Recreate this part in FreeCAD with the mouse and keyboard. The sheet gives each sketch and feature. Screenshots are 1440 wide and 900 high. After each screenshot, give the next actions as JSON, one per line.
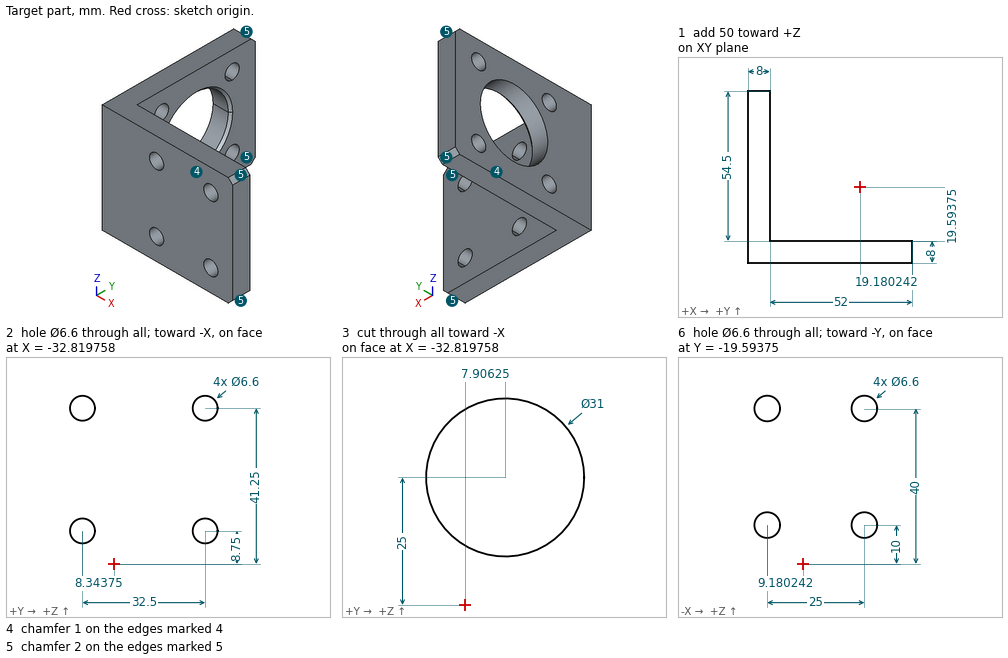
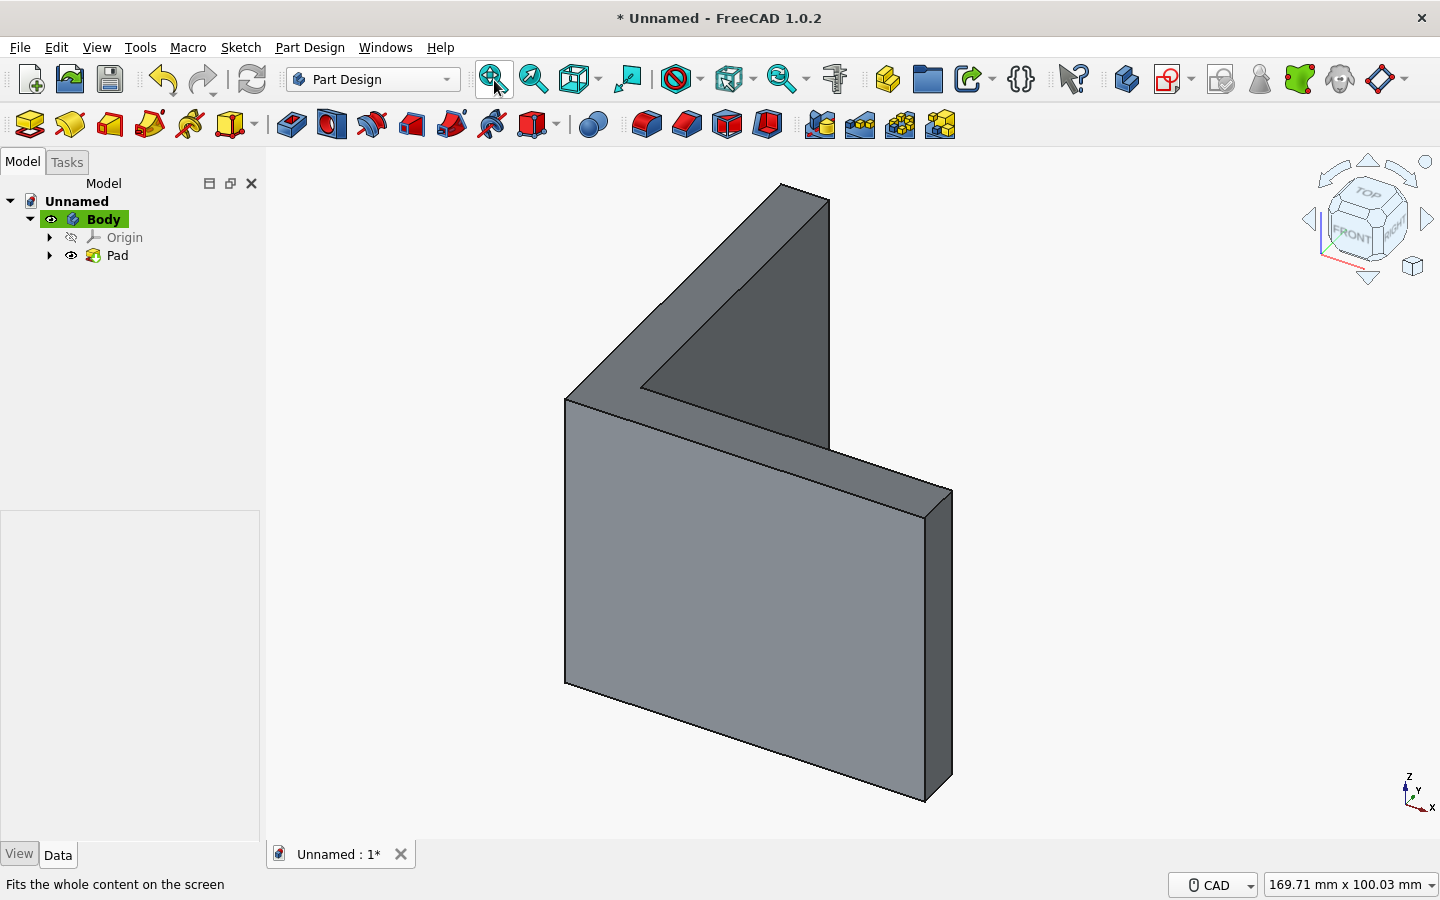
{"action": "left_click", "coordinate": [762, 408]}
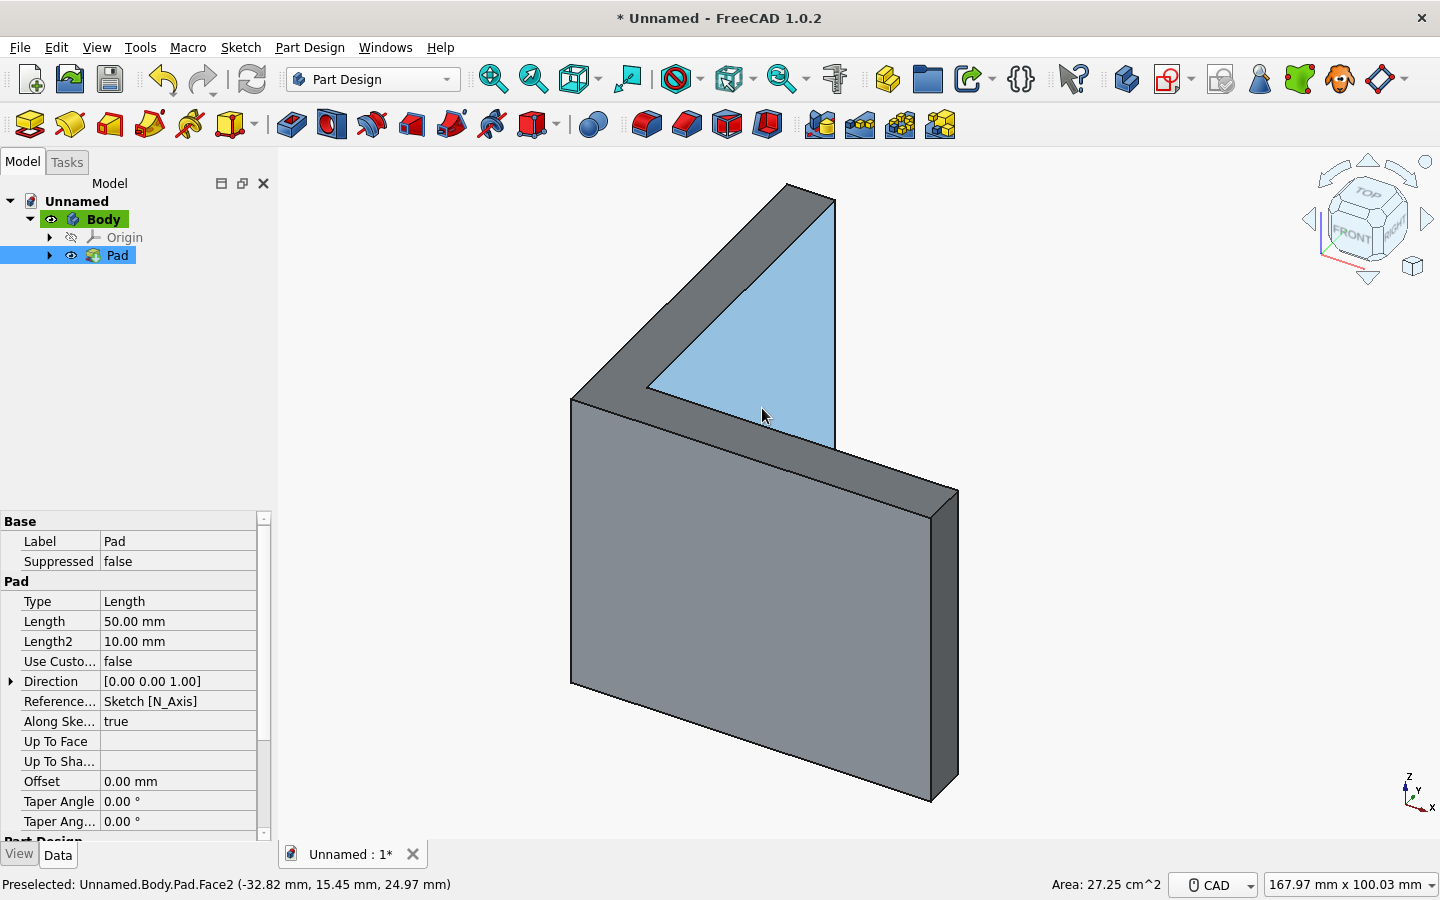
{"action": "left_click", "coordinate": [1168, 80]}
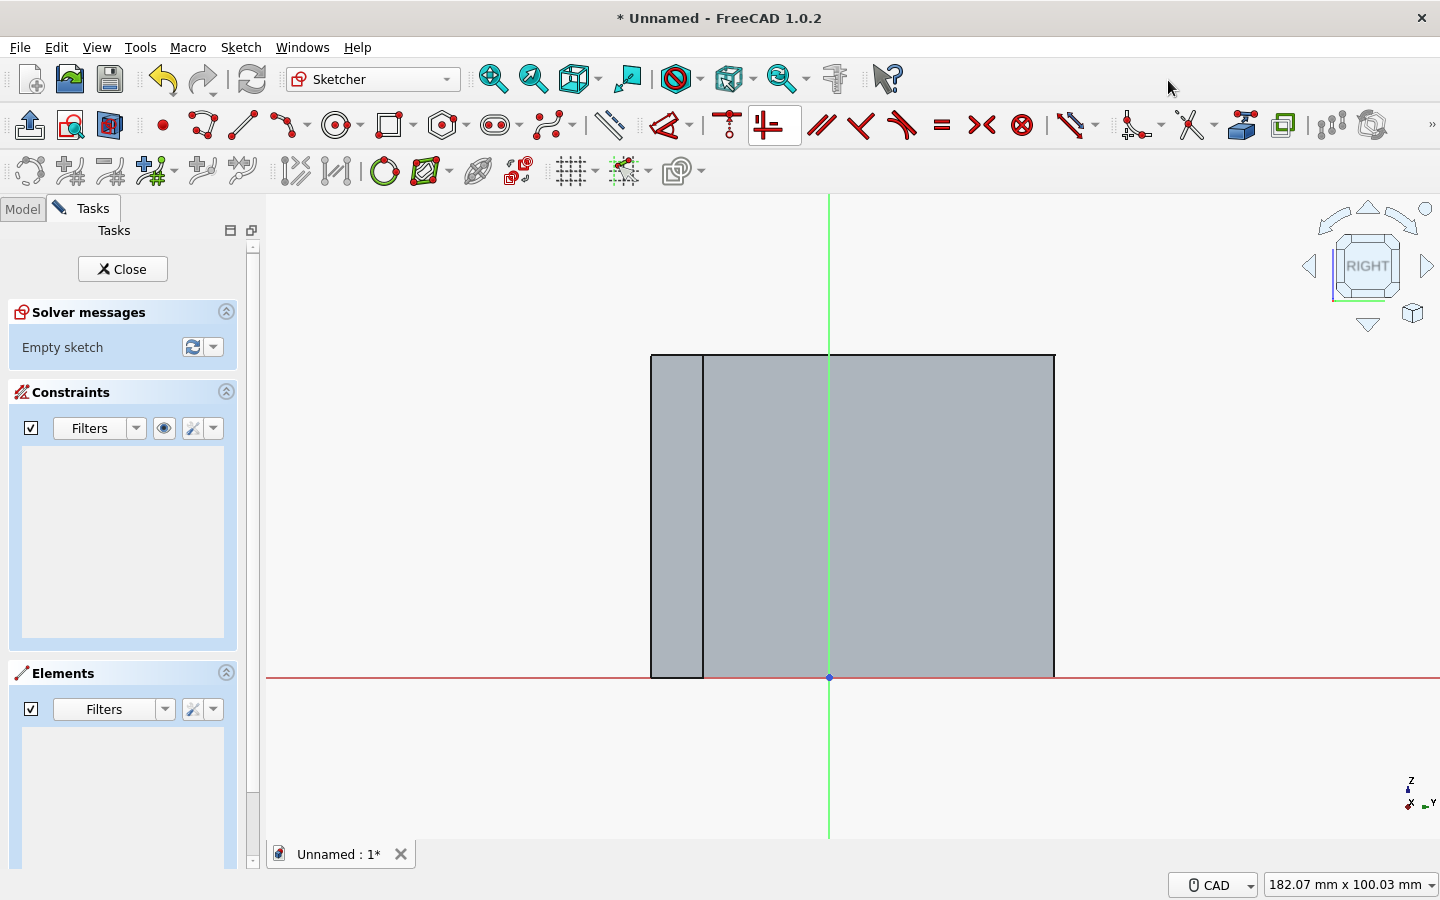
{"action": "scroll", "coordinate": [1075, 570], "scroll_direction": "up", "scroll_amount": 2}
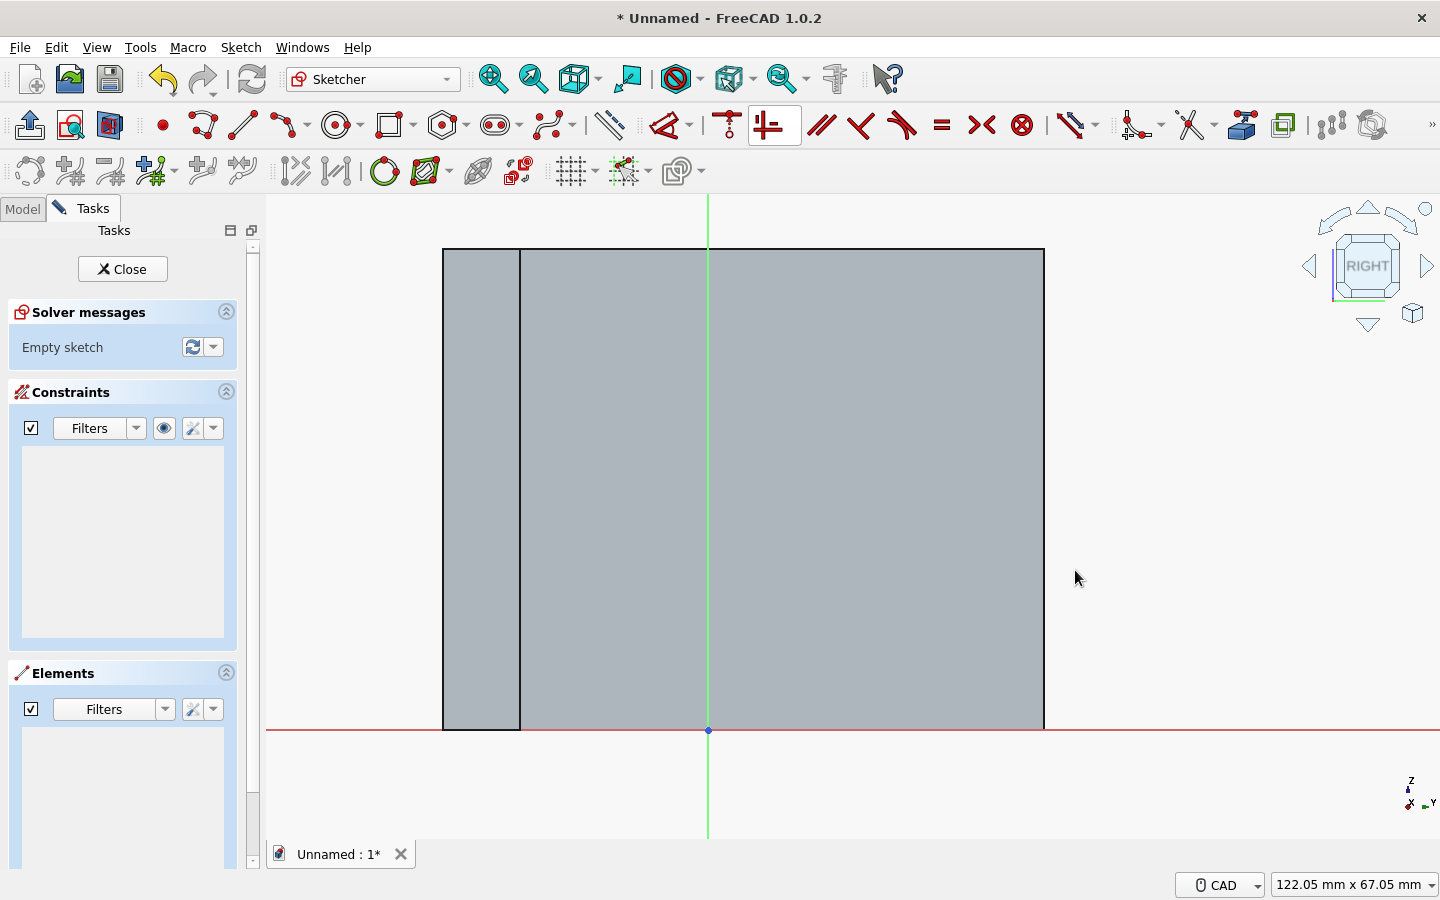
{"action": "left_click", "coordinate": [336, 126]}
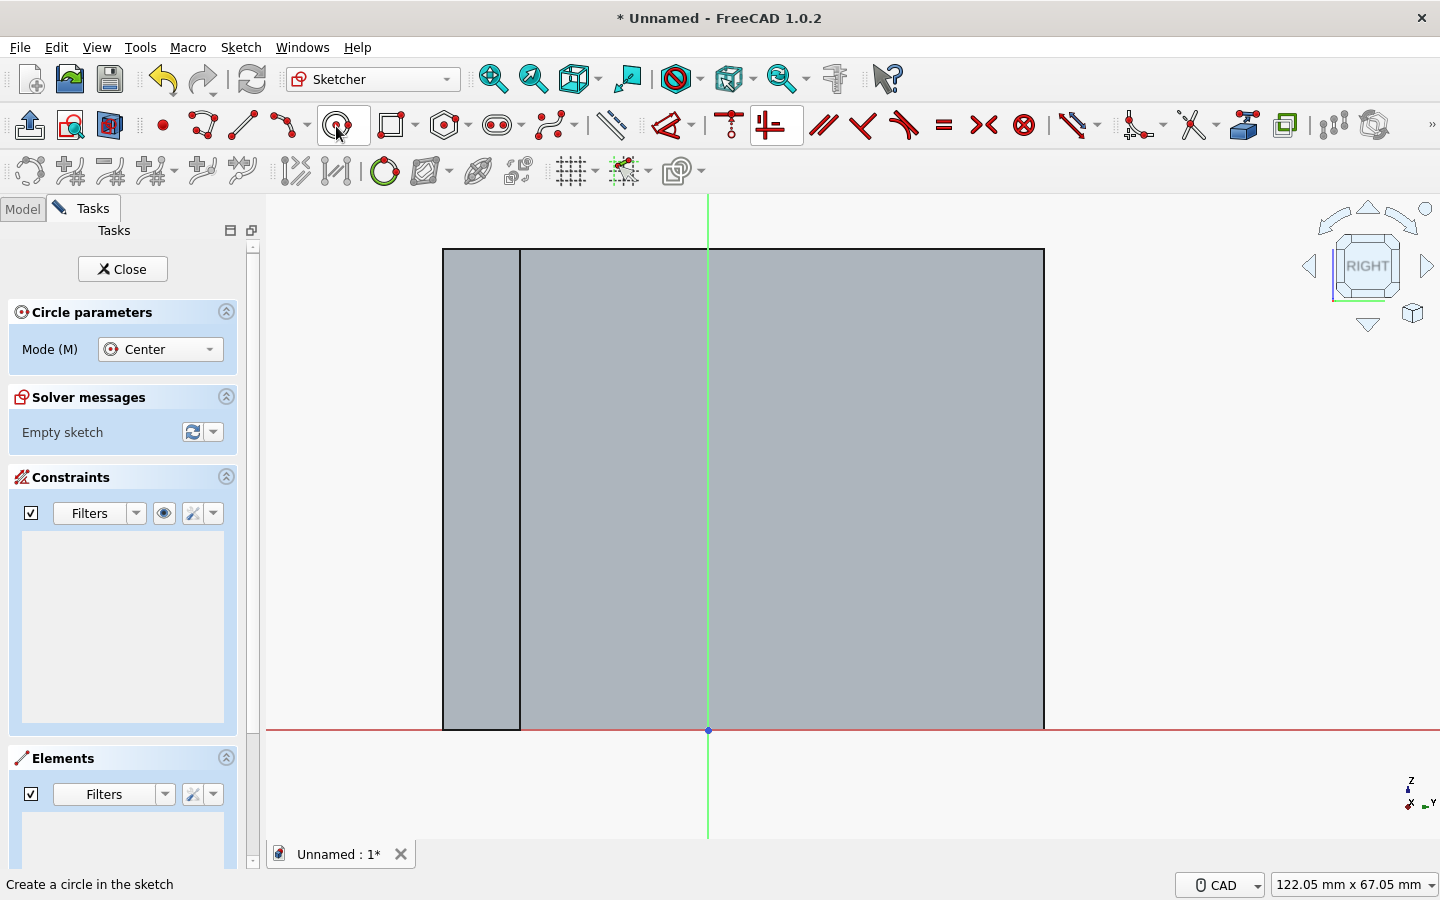
{"action": "left_click", "coordinate": [941, 334]}
{"action": "mouse_move", "coordinate": [963, 311]}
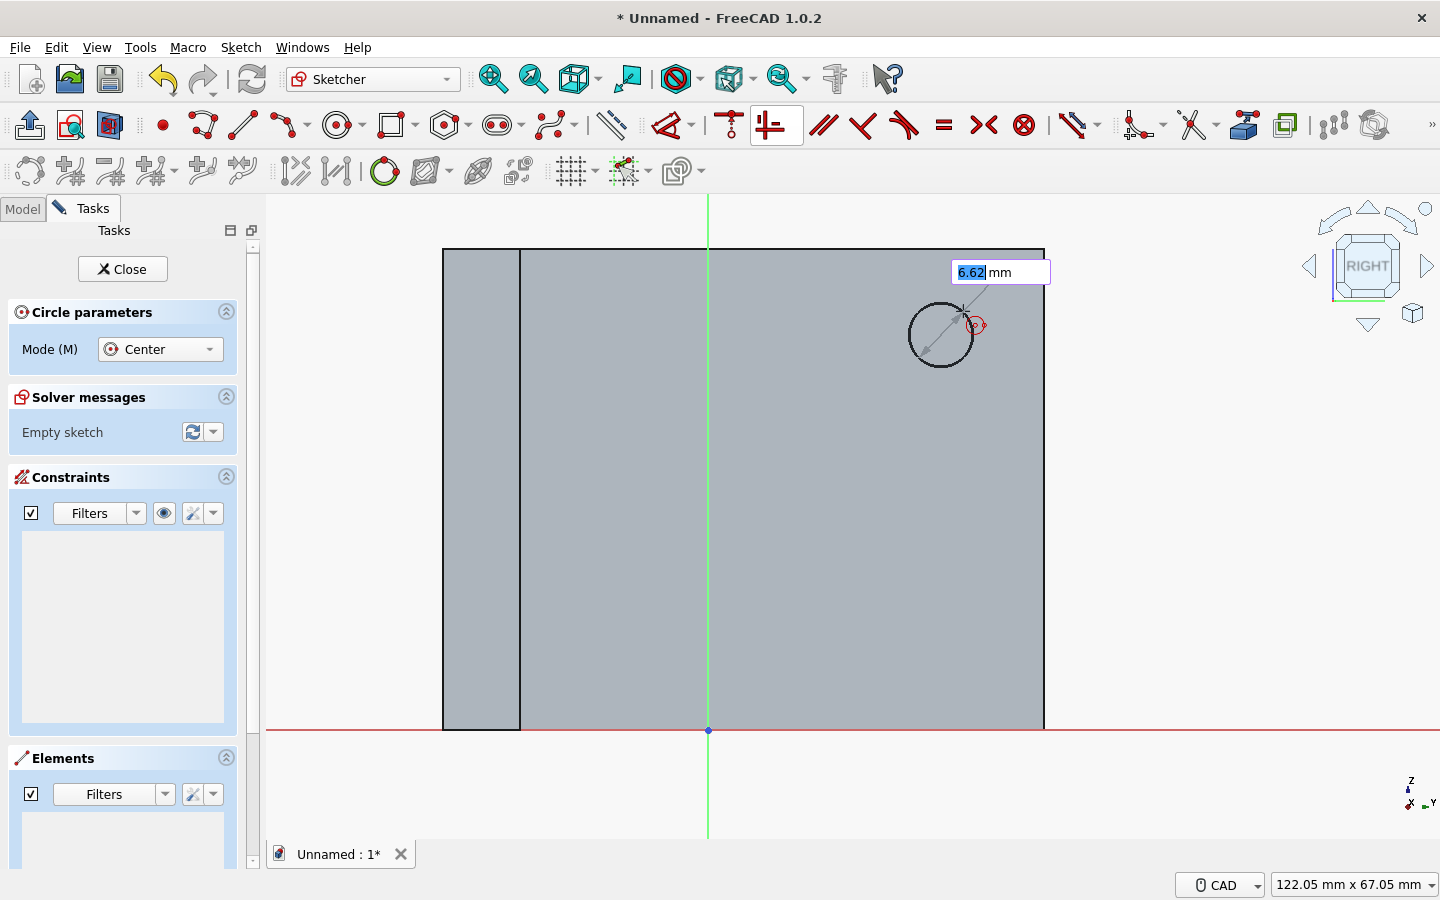
{"action": "type", "text": "6.6"}
{"action": "key", "text": "Return"}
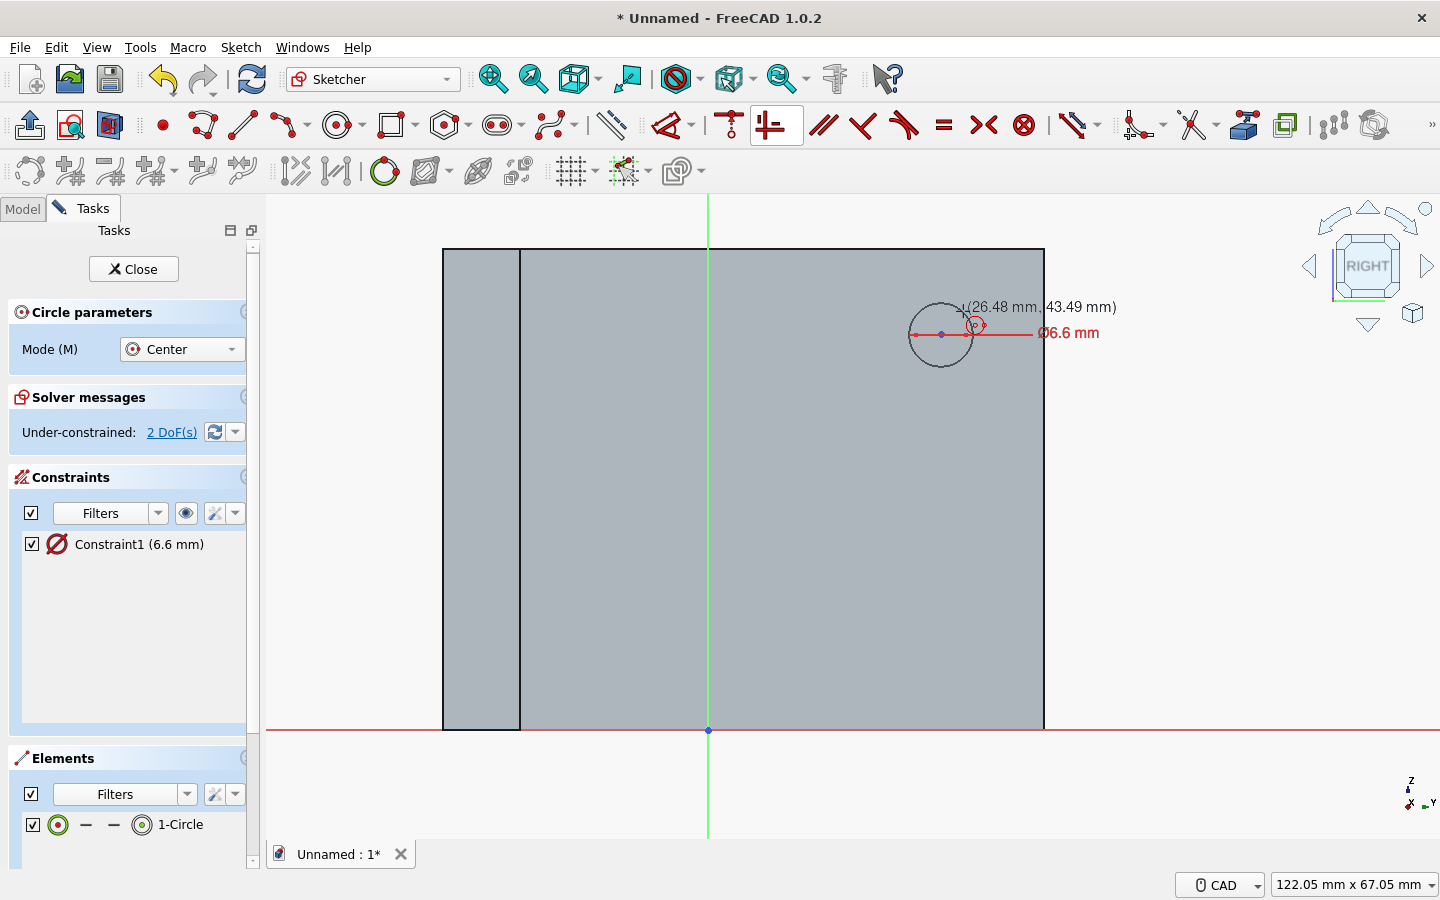
{"action": "left_click", "coordinate": [941, 646]}
{"action": "mouse_move", "coordinate": [963, 624]}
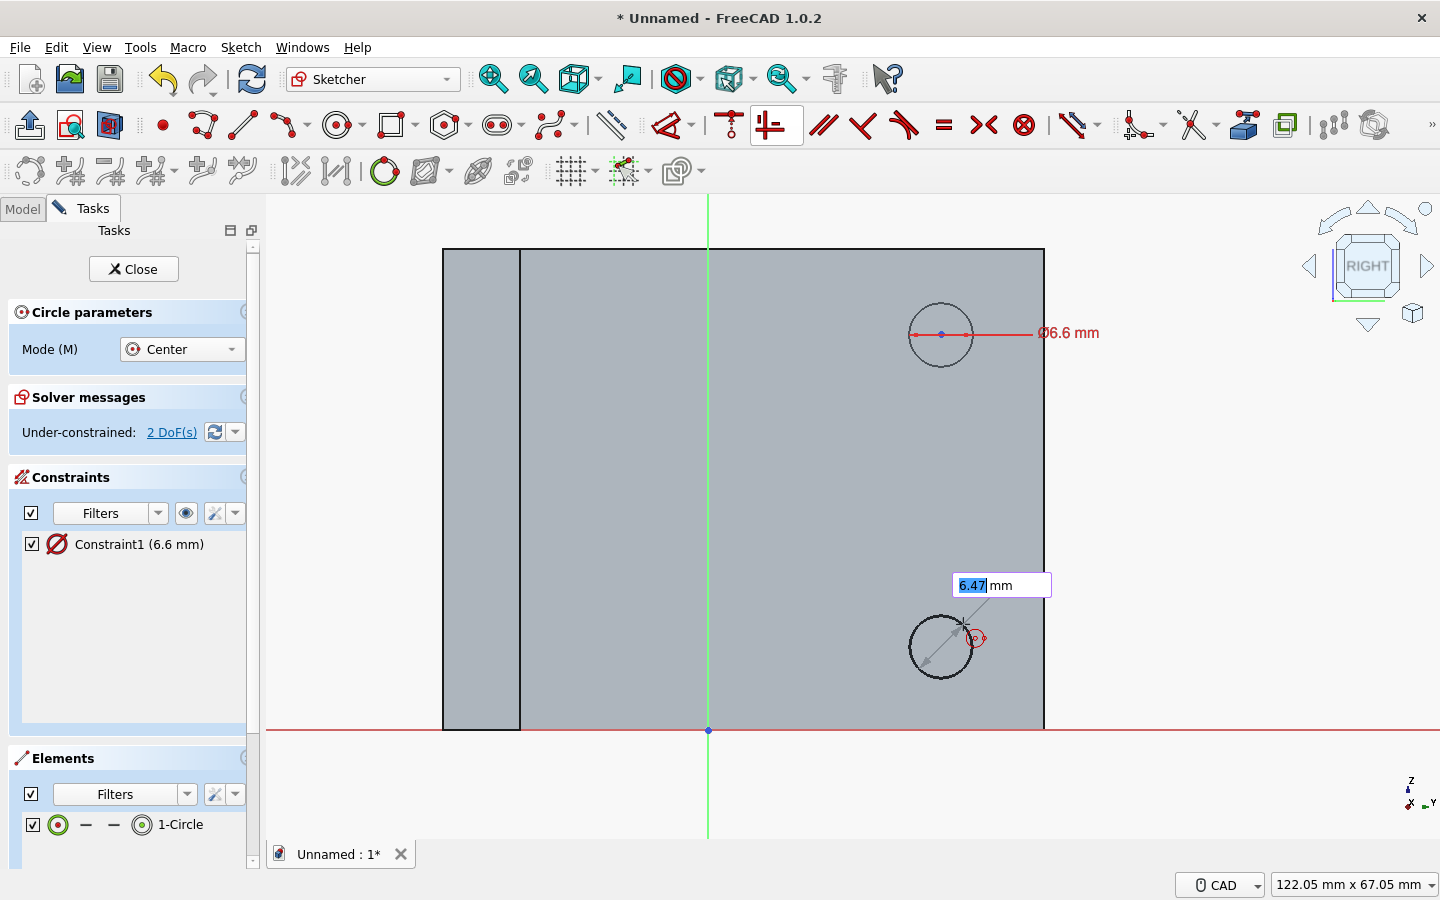
{"action": "type", "text": "6.6"}
{"action": "key", "text": "Return"}